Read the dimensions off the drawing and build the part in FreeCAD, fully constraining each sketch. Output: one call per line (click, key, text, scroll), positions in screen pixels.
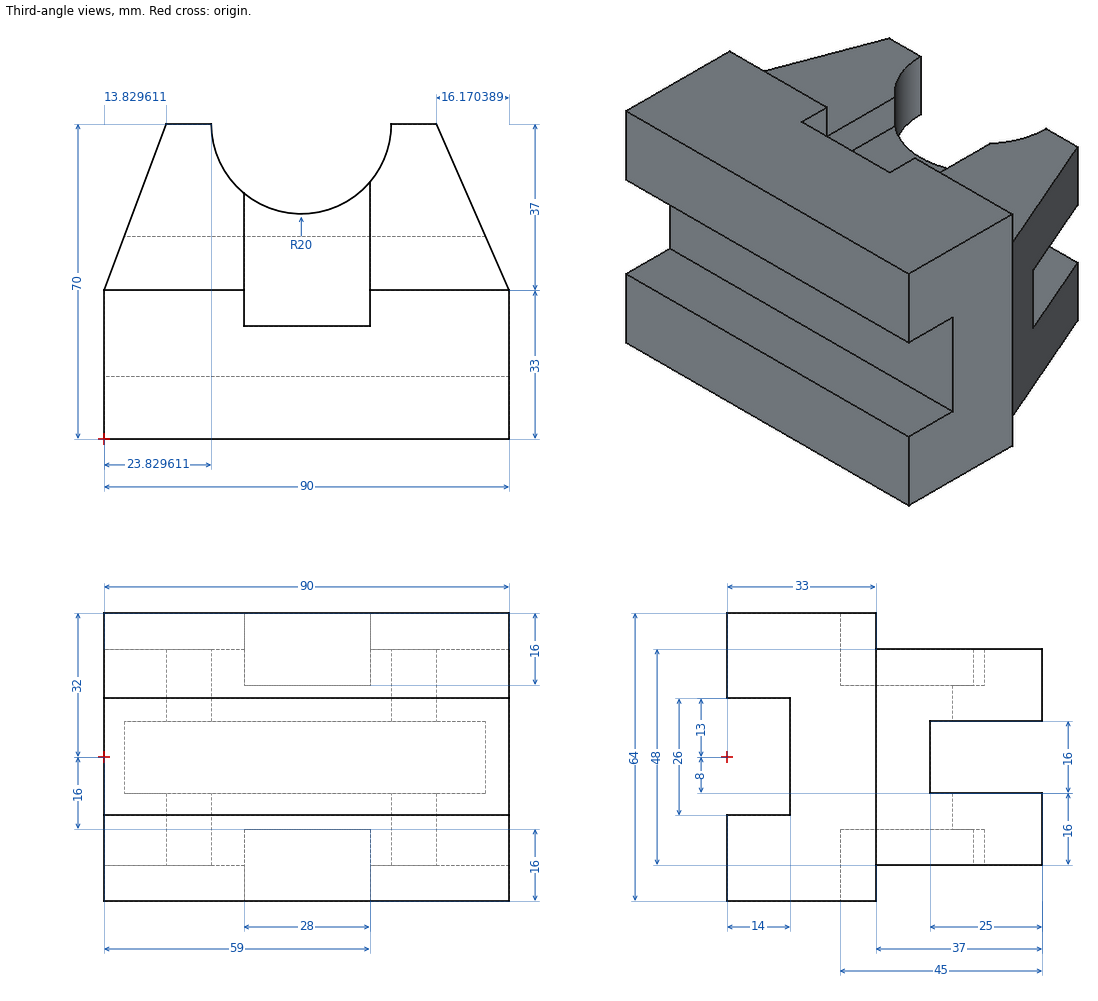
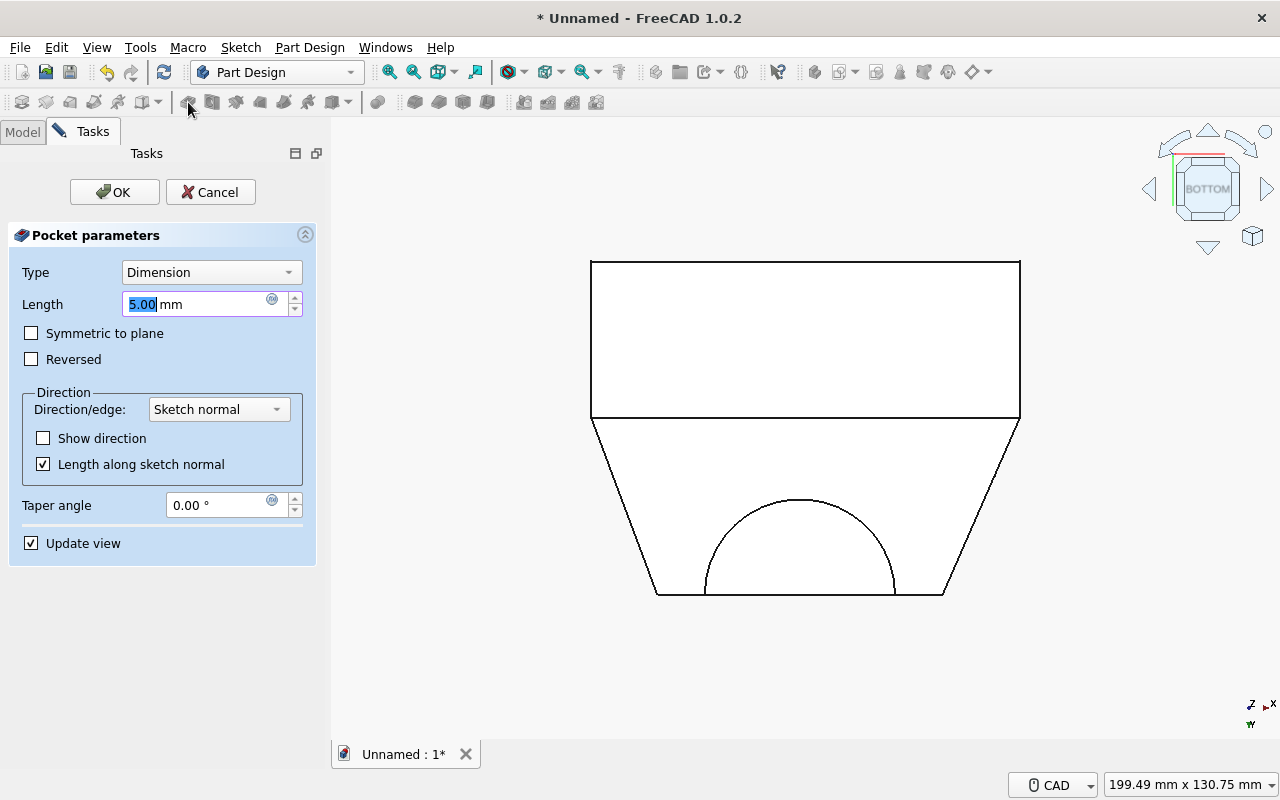
click(212, 272)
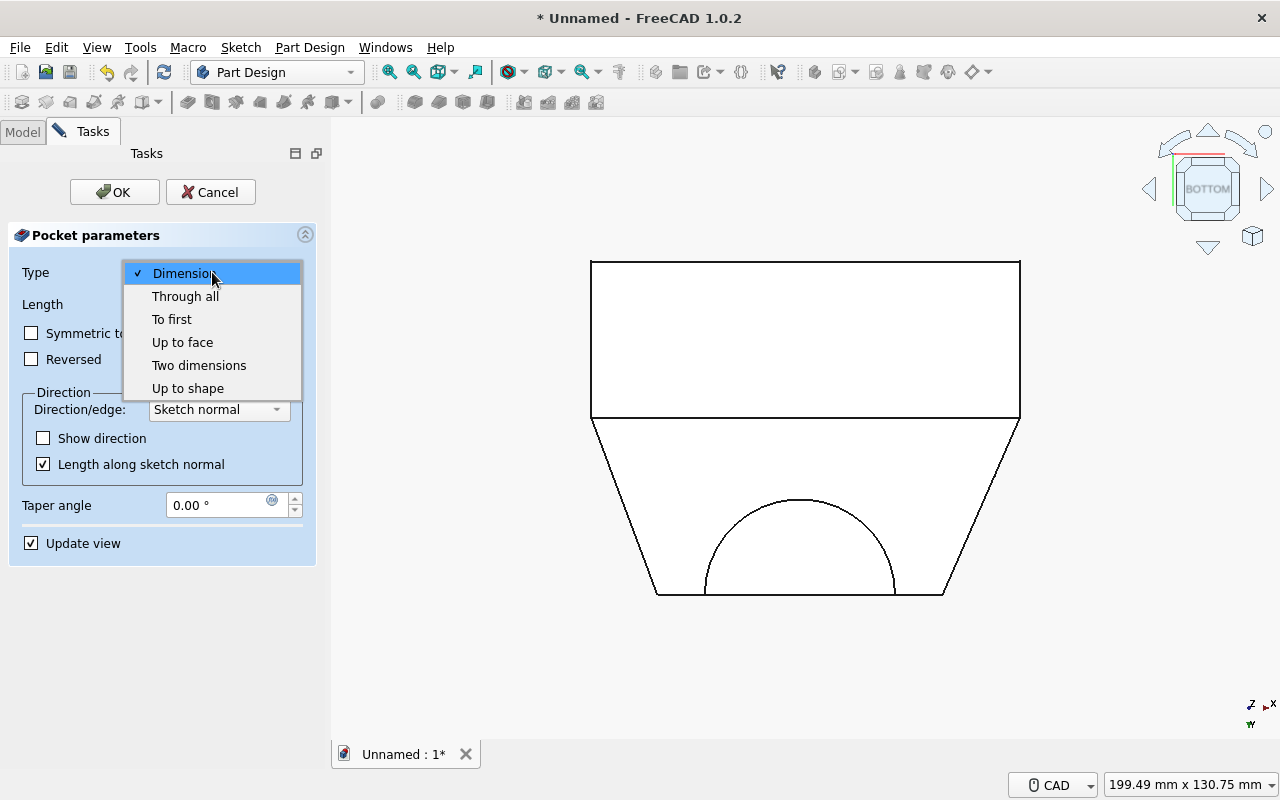
click(212, 296)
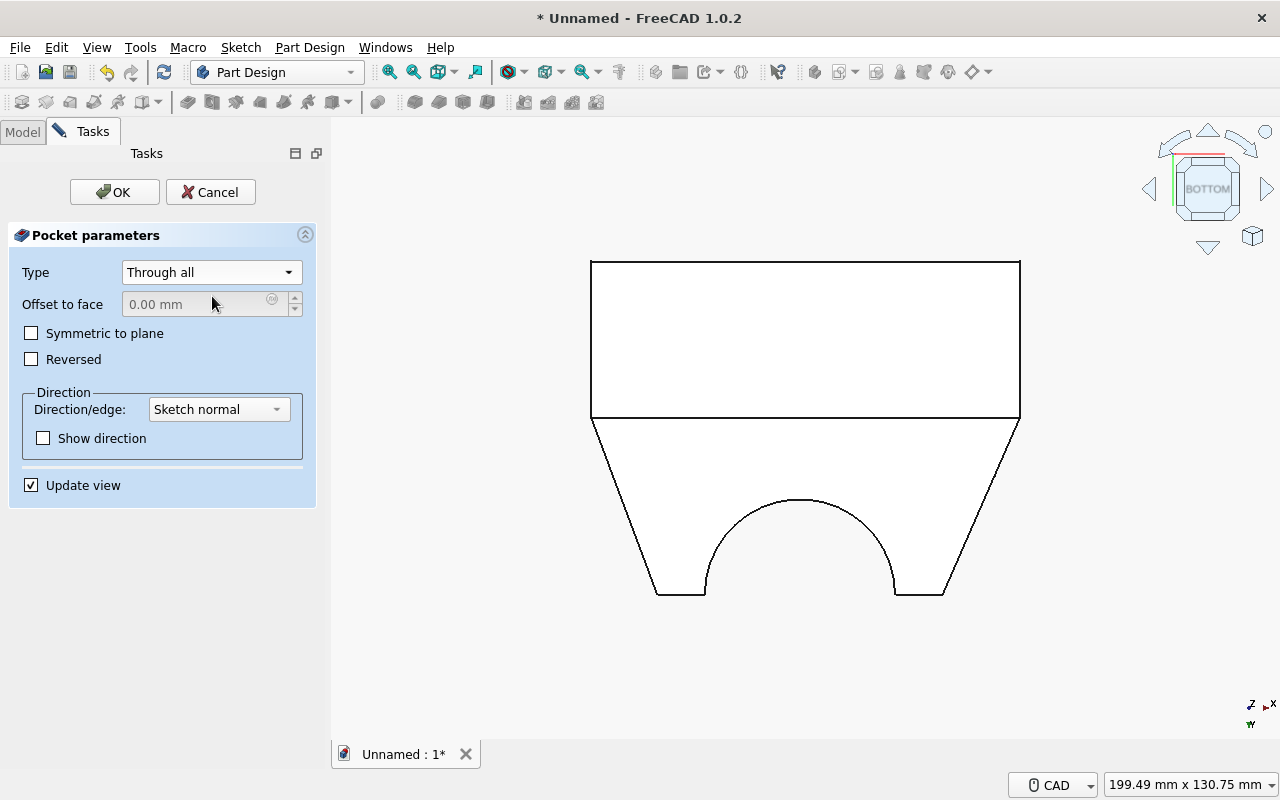
click(115, 192)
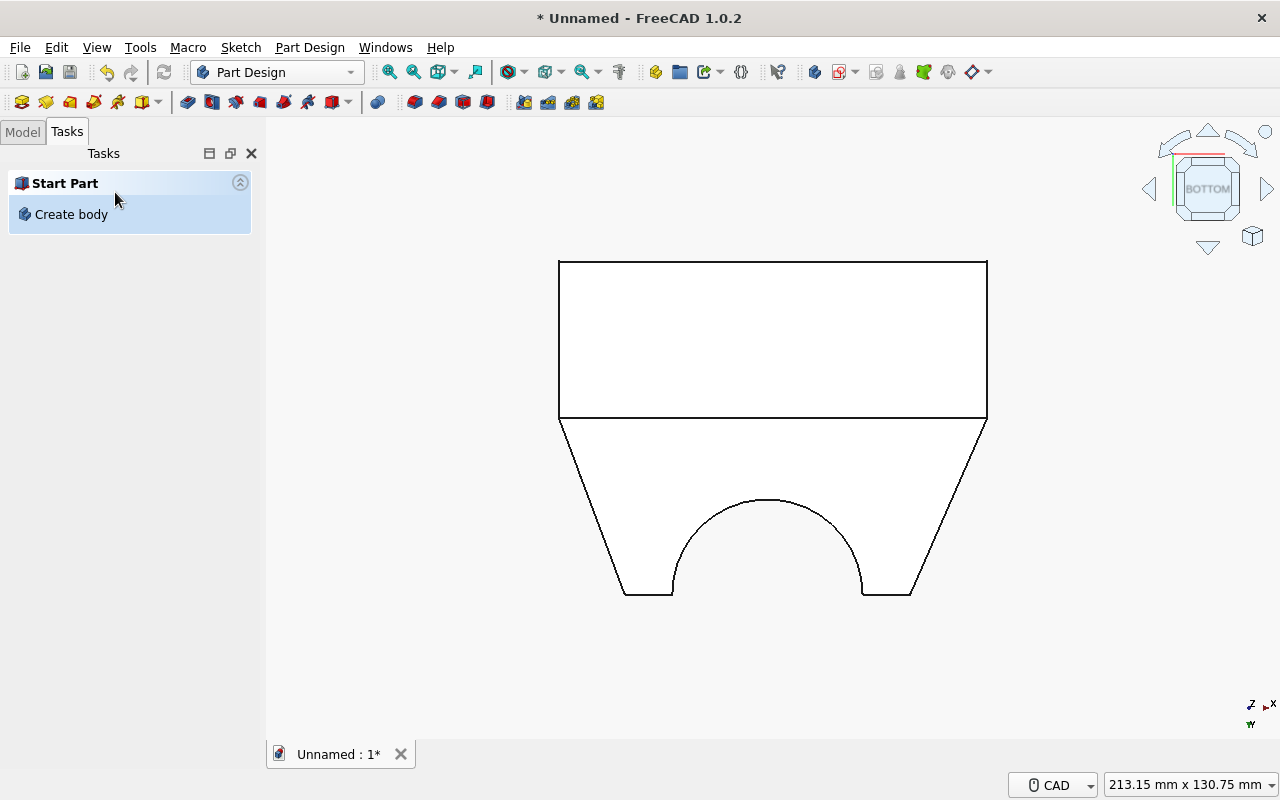
key(4)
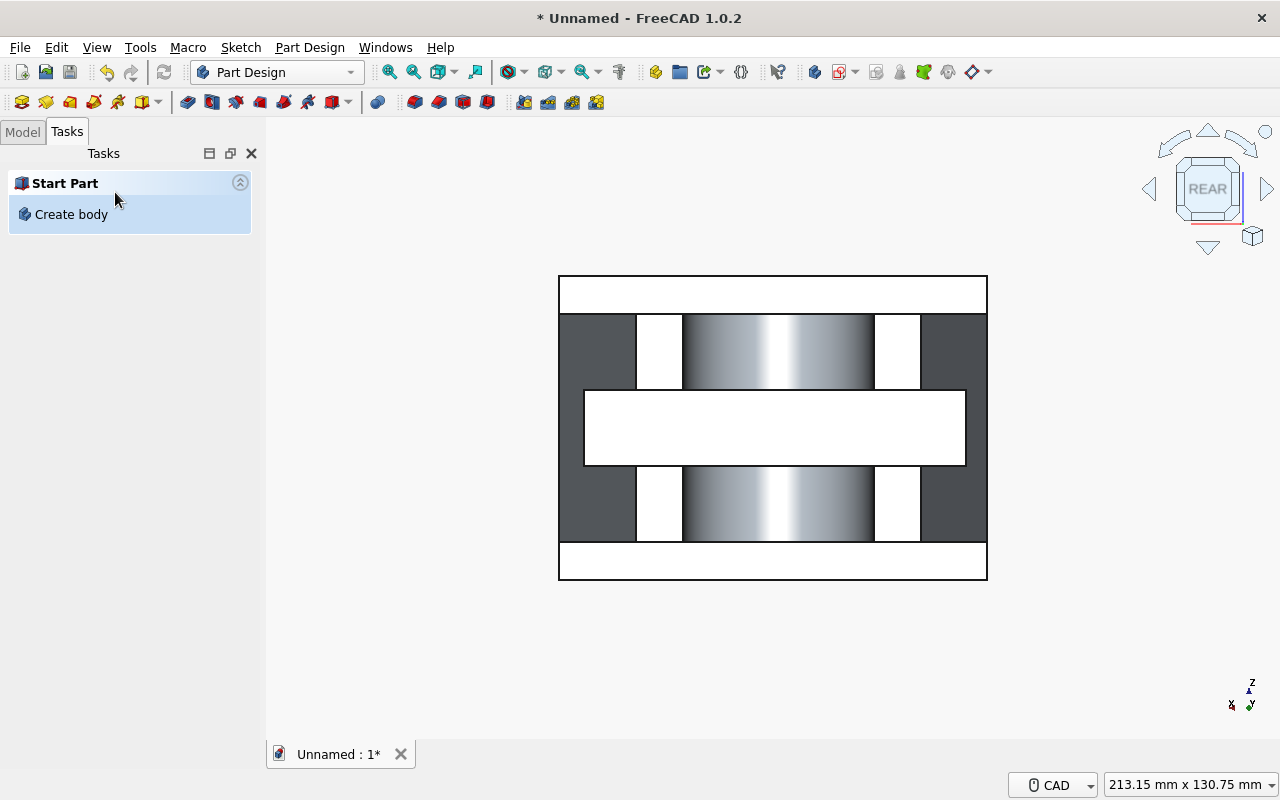
click(897, 340)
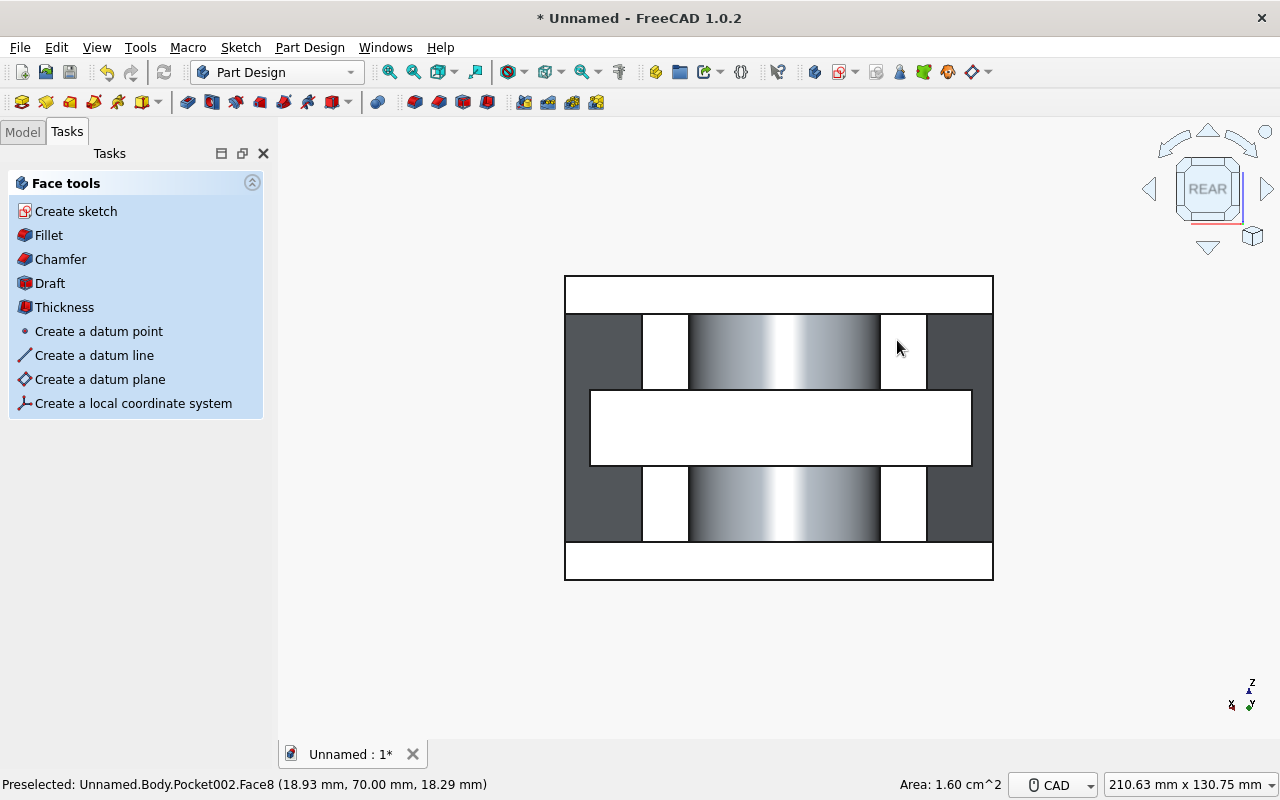
click(840, 72)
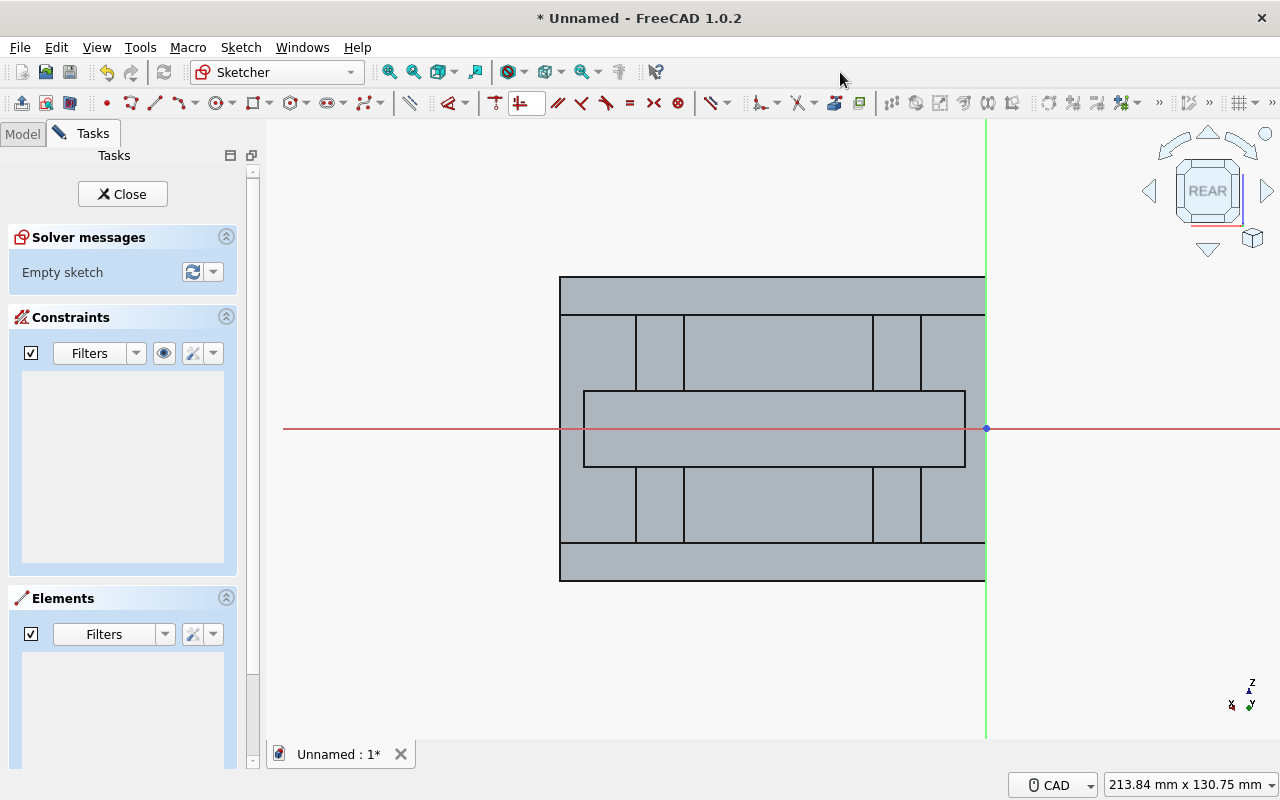
click(254, 104)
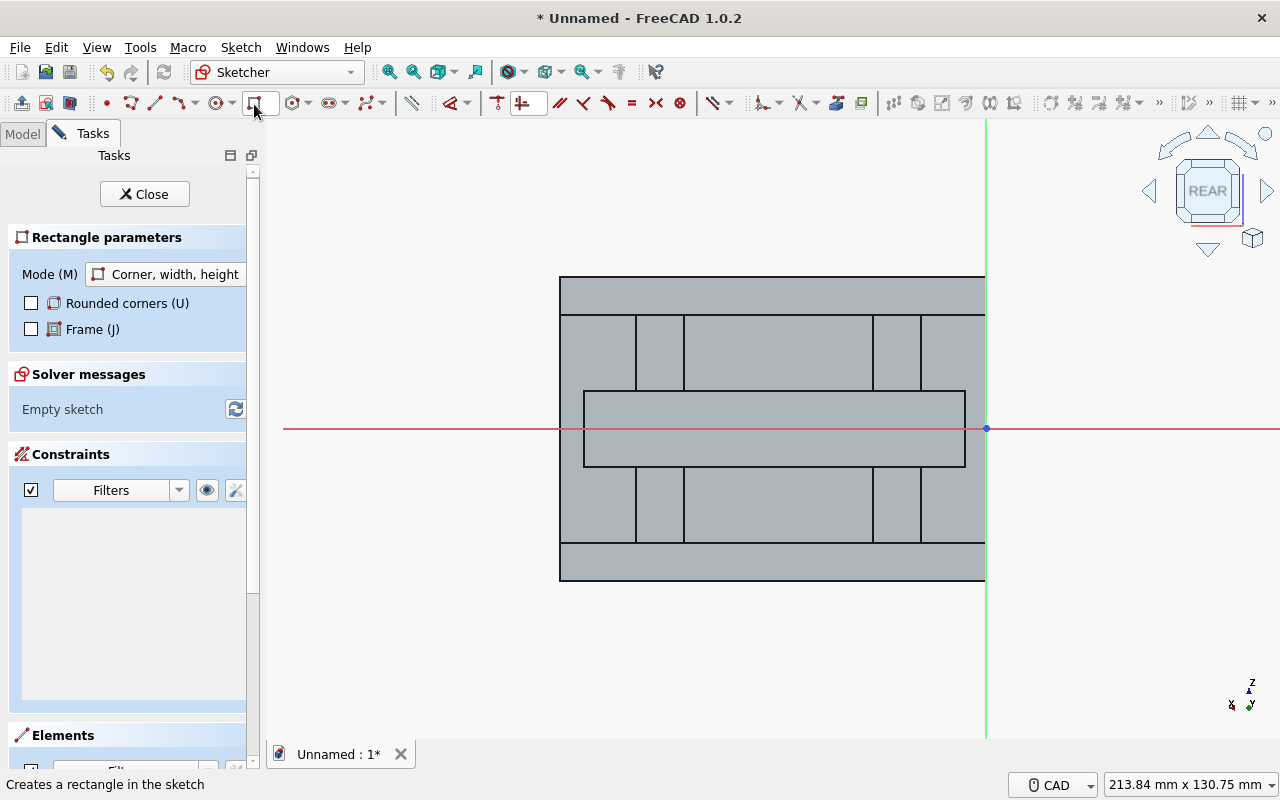
click(707, 505)
click(839, 581)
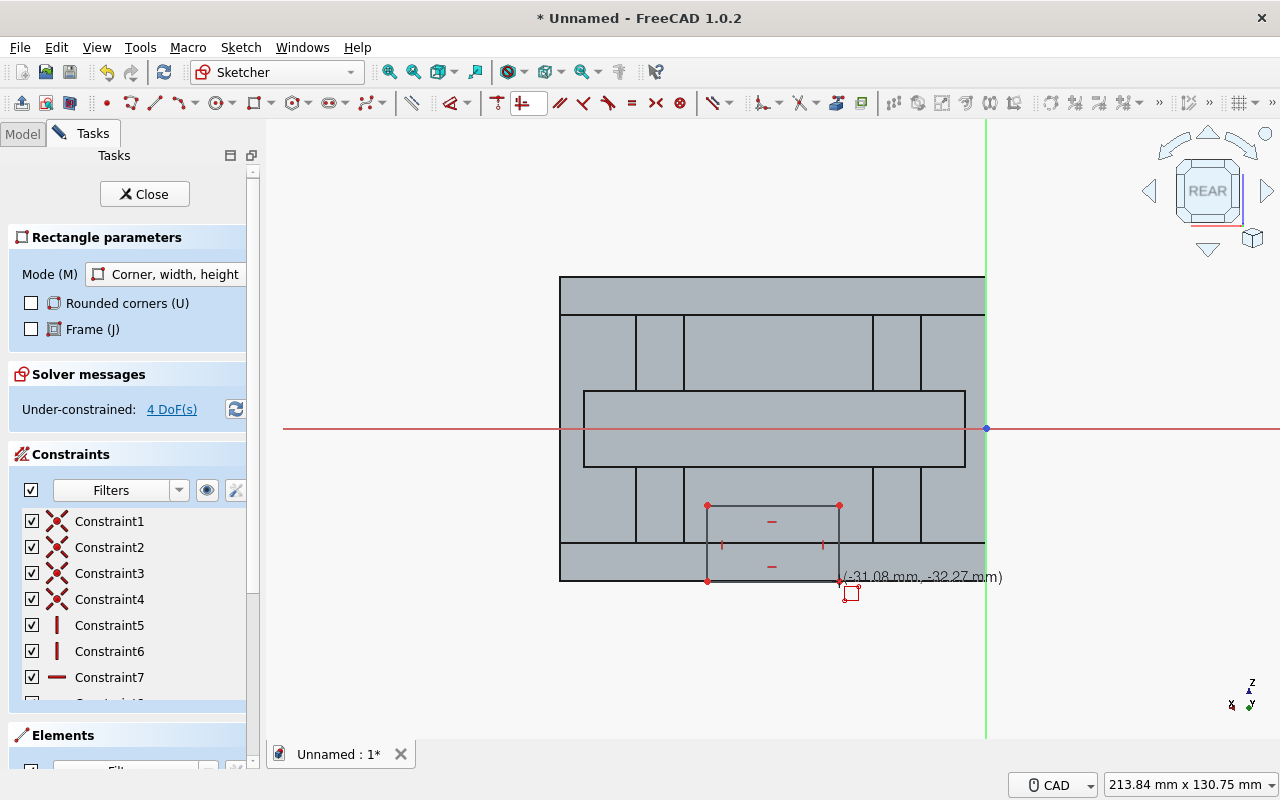
click(707, 277)
click(839, 353)
key(Escape)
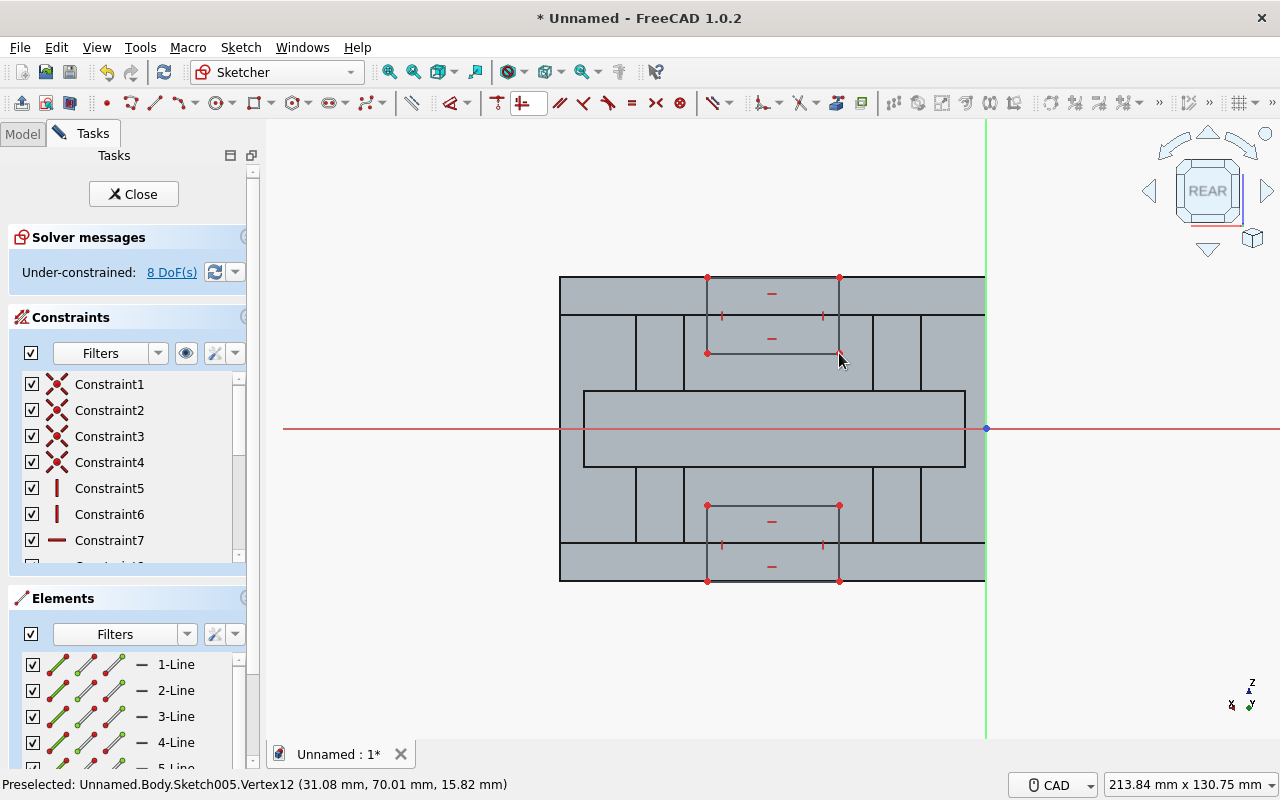
click(450, 104)